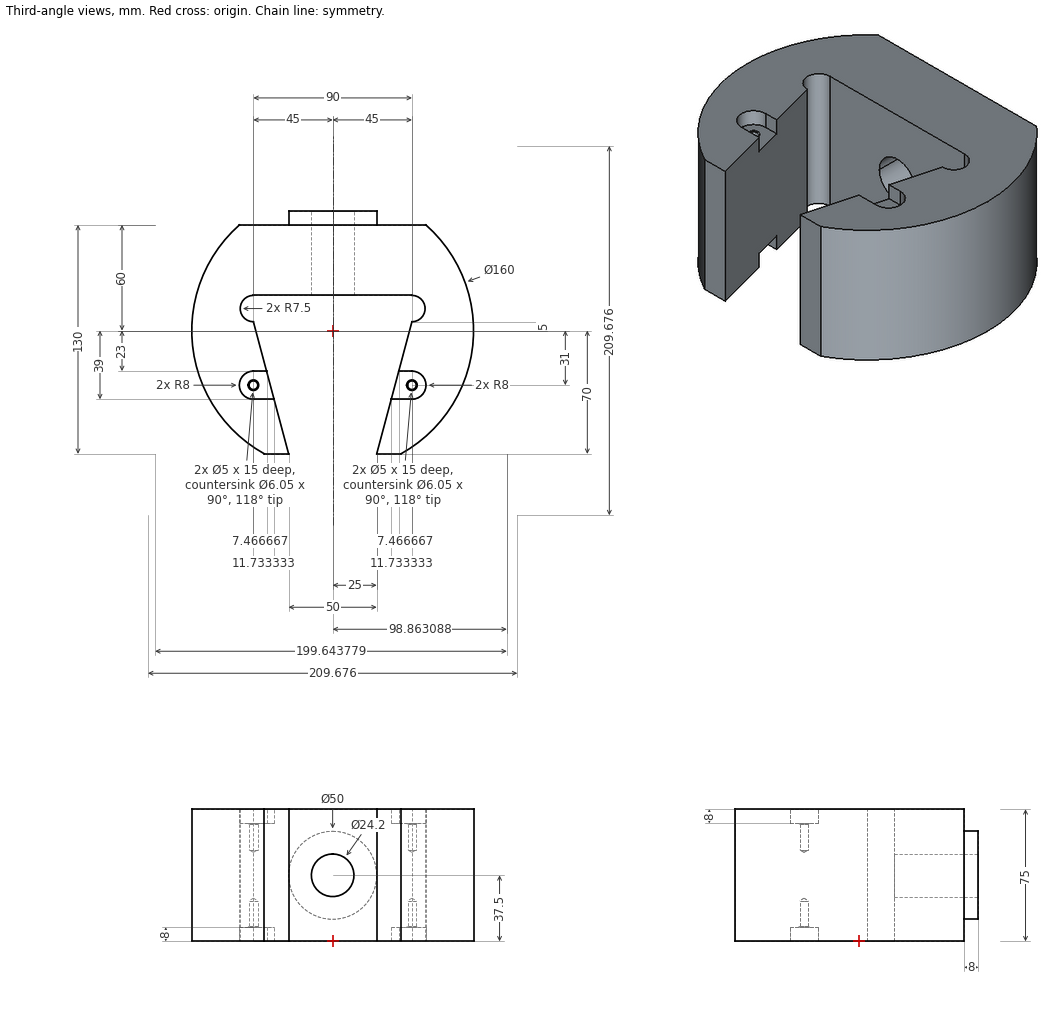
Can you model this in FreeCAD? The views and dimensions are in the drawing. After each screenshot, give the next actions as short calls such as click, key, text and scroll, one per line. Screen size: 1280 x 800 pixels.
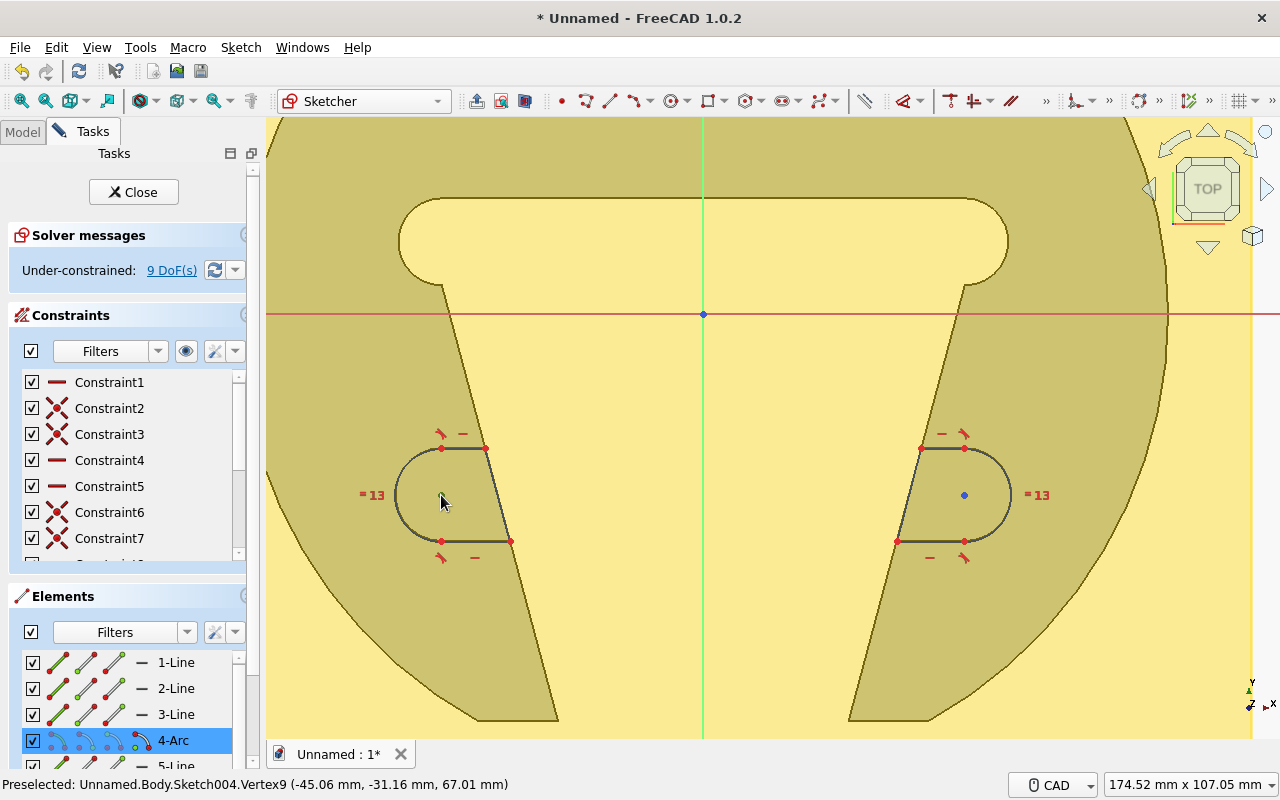
click(964, 495)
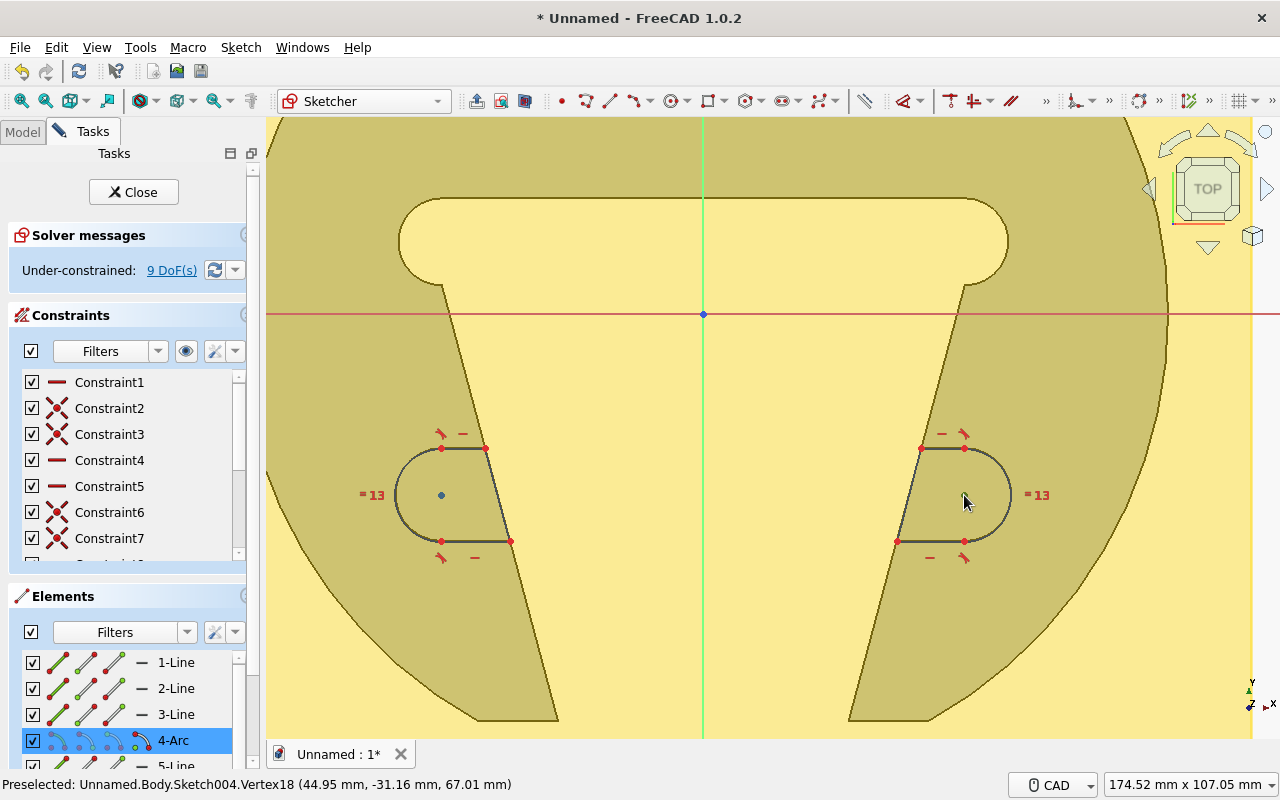
click(703, 671)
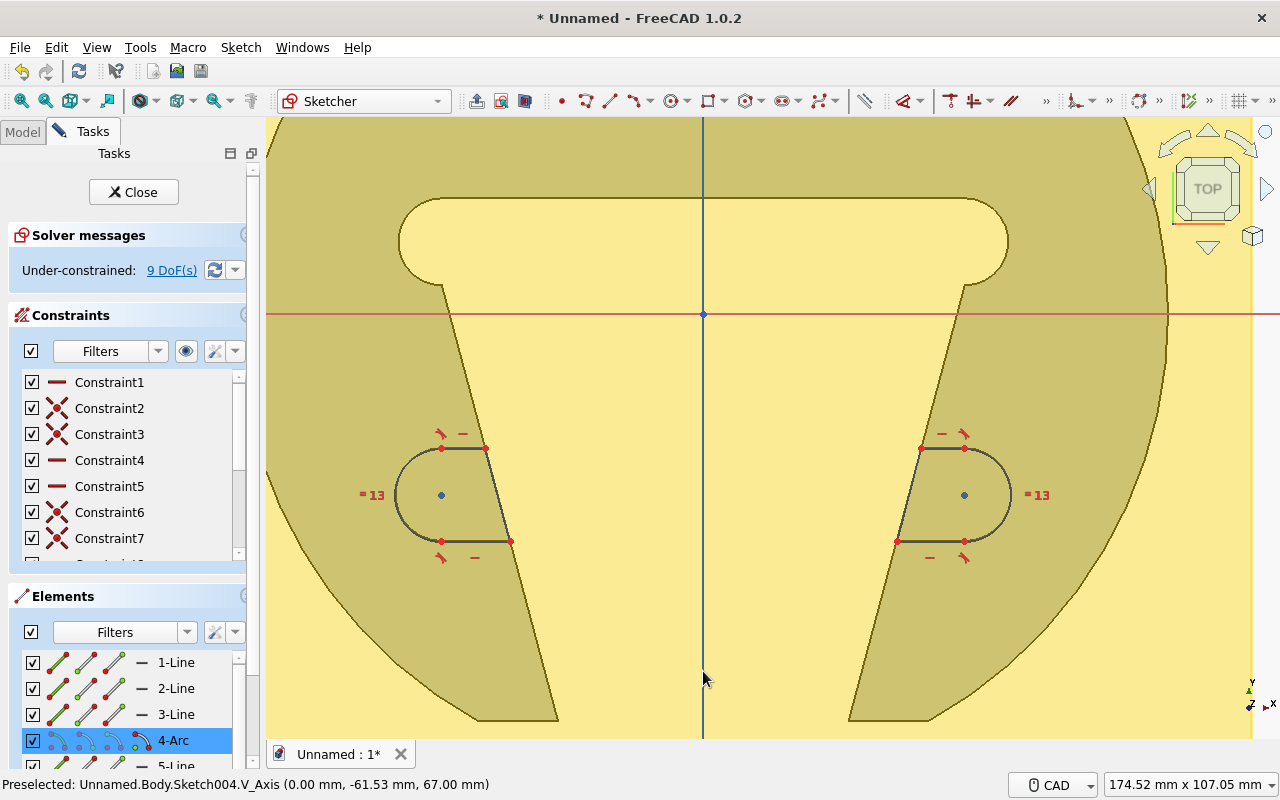
key(s)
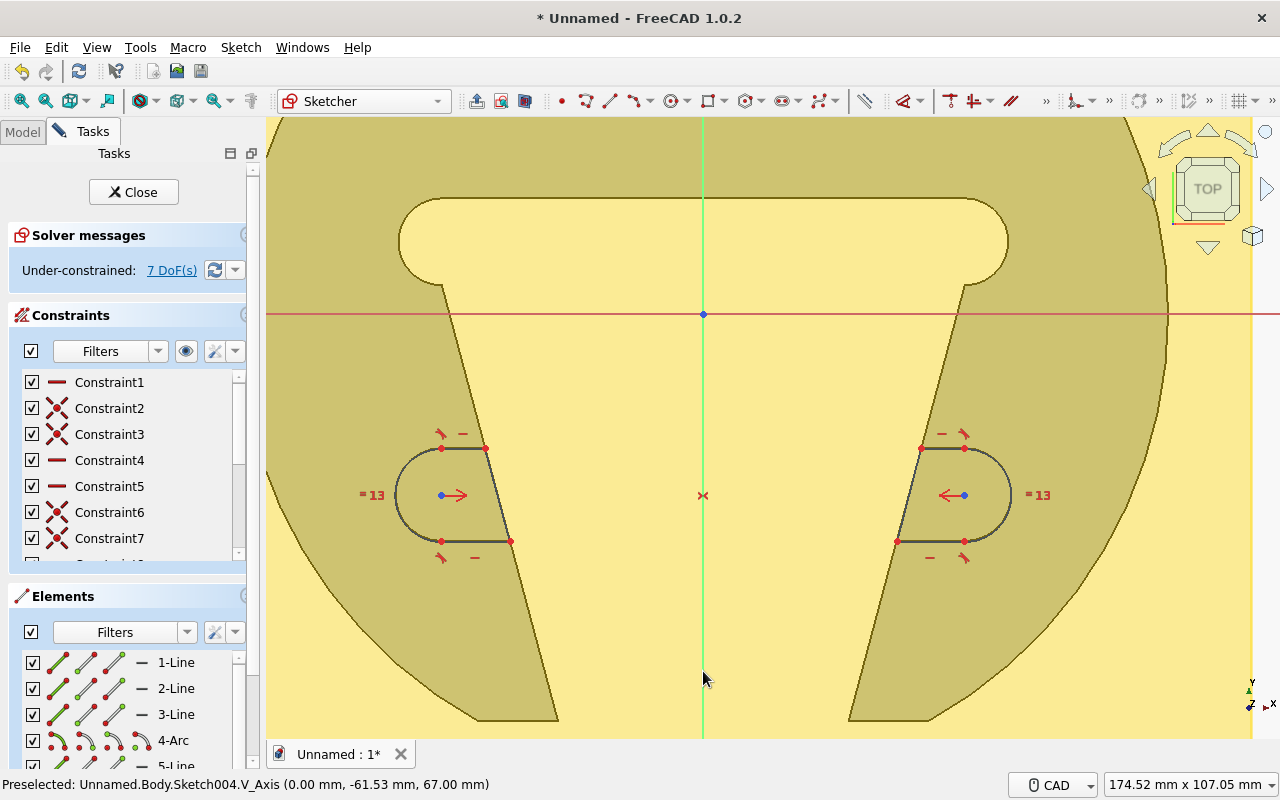
key(d)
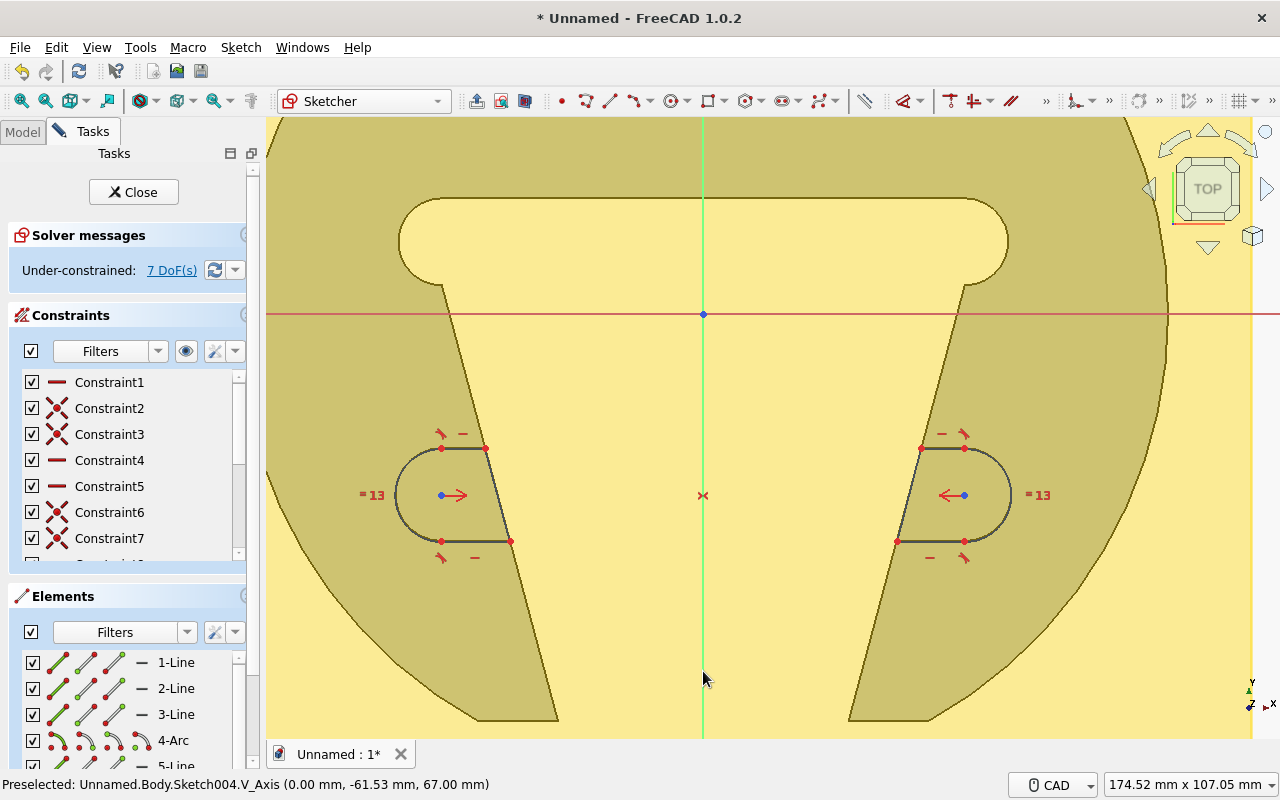
click(404, 468)
click(378, 449)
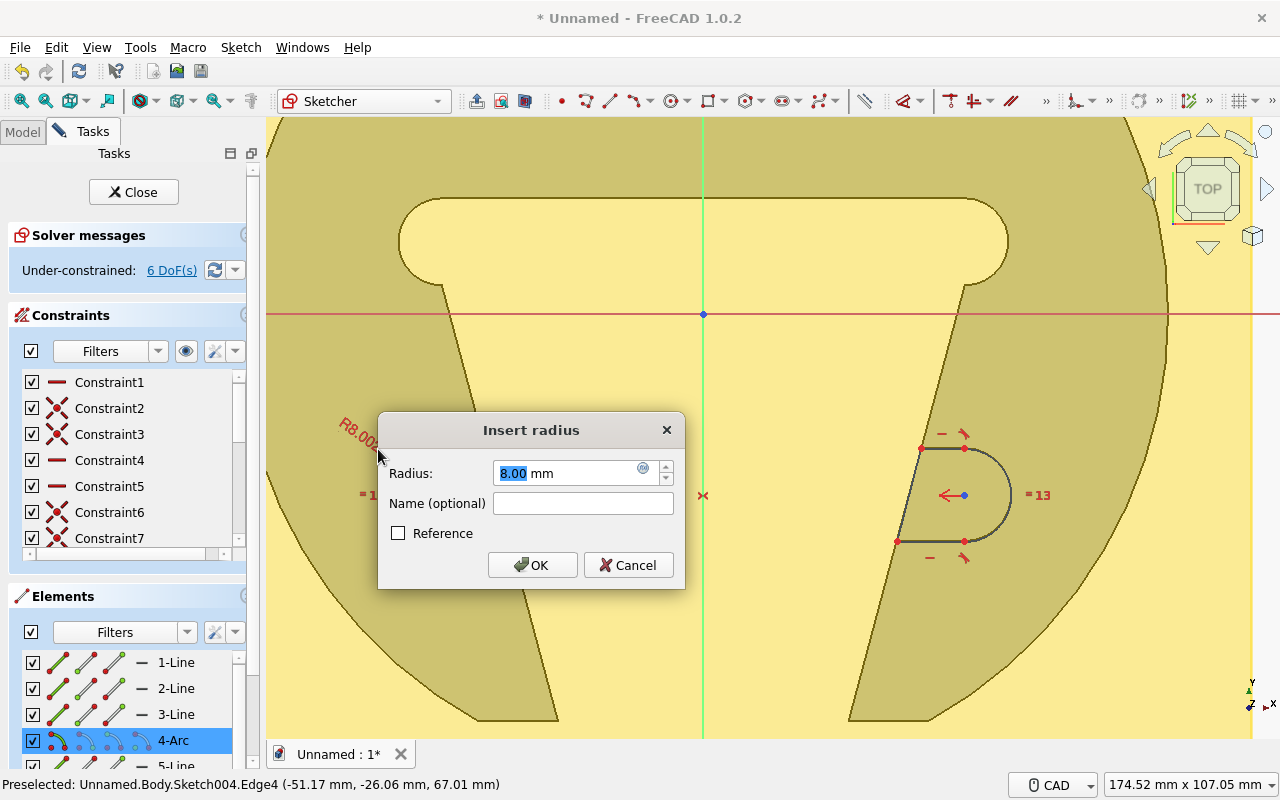
text(8)
key(Return)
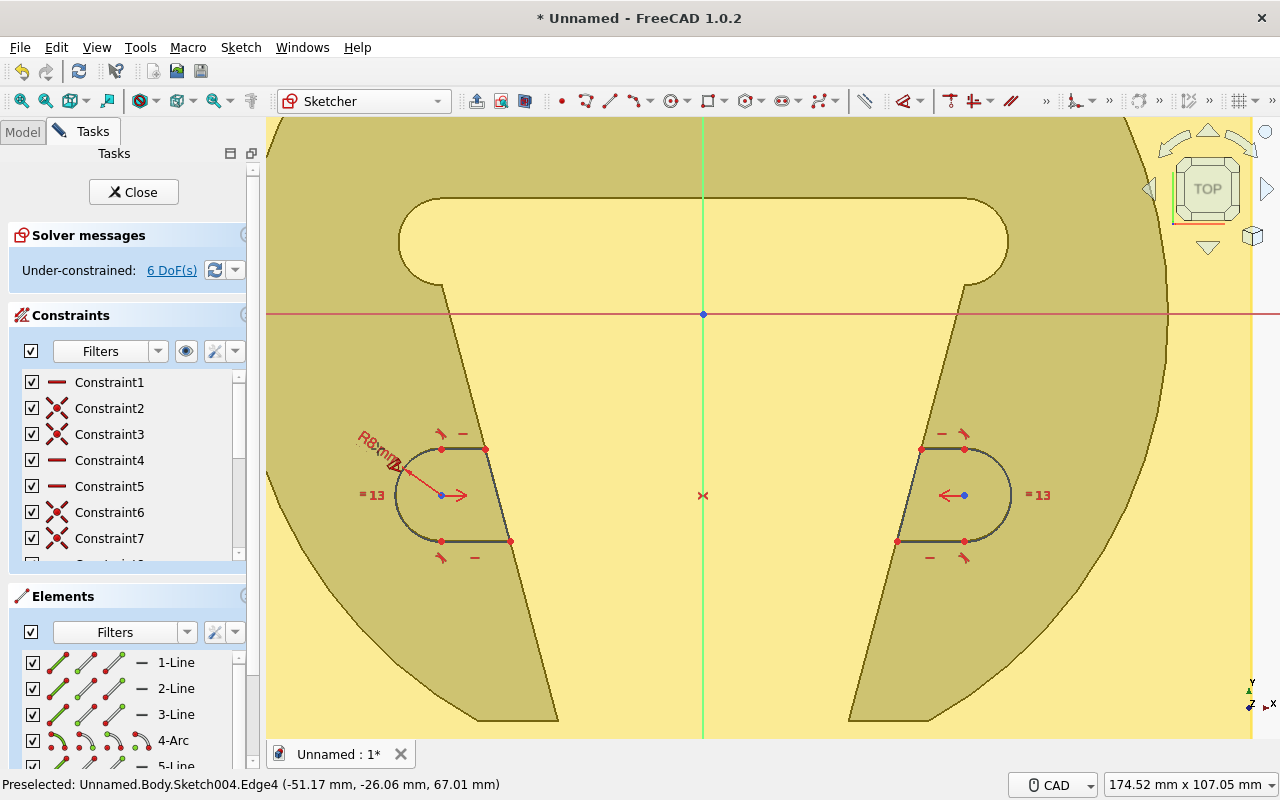
click(442, 449)
click(573, 280)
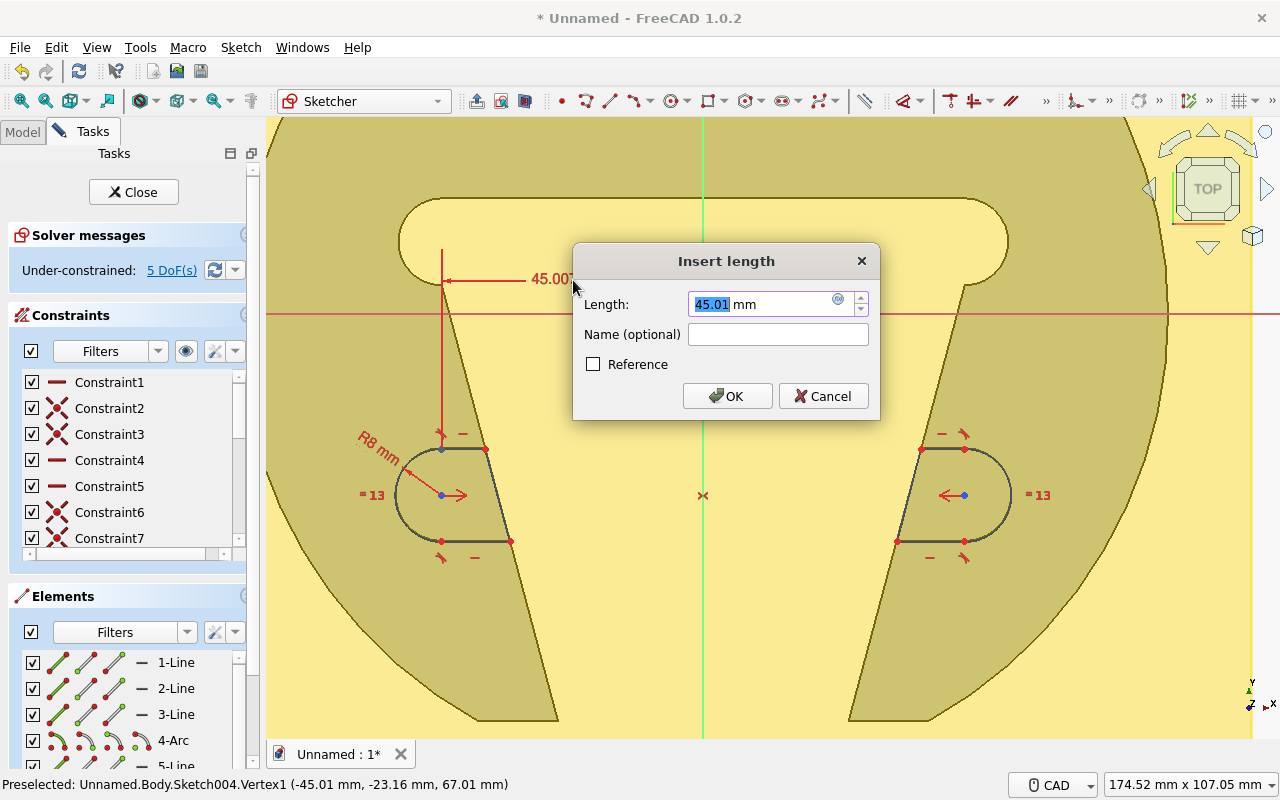
text(45)
key(Return)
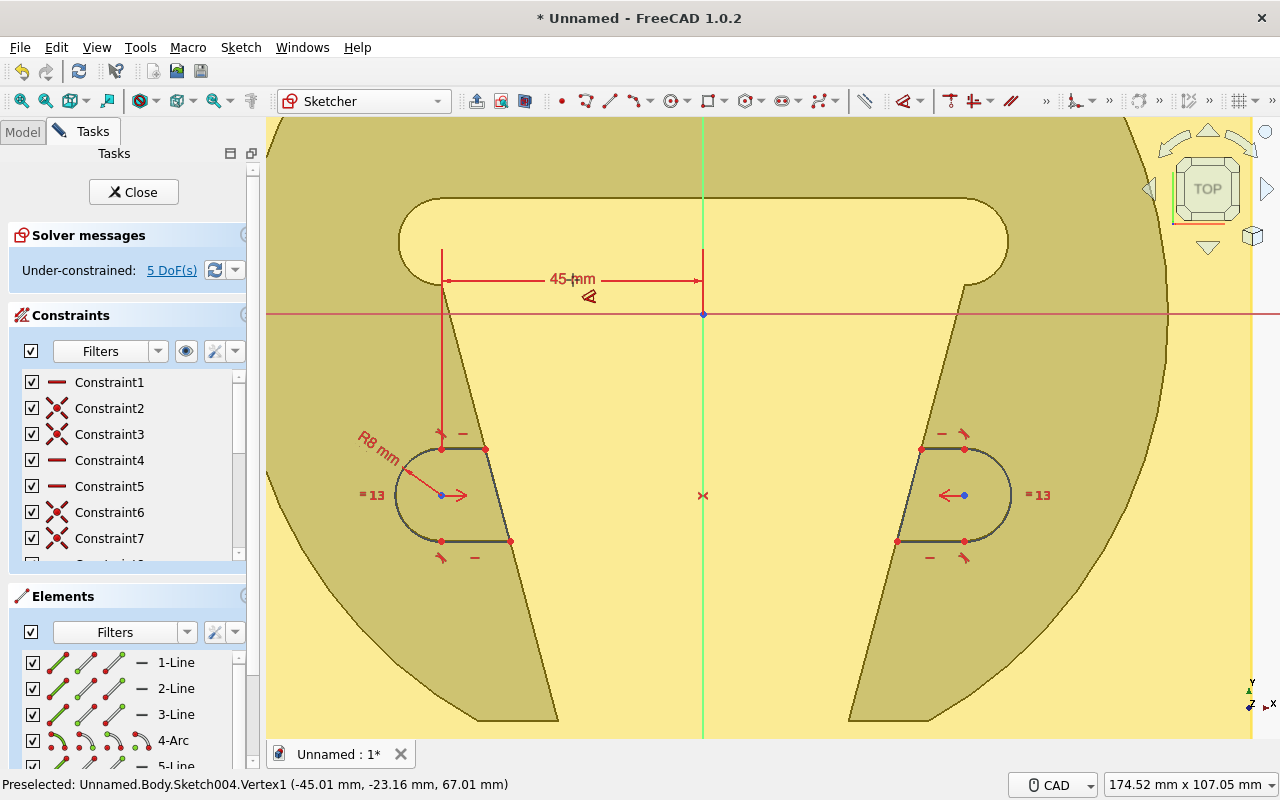
click(442, 449)
click(408, 382)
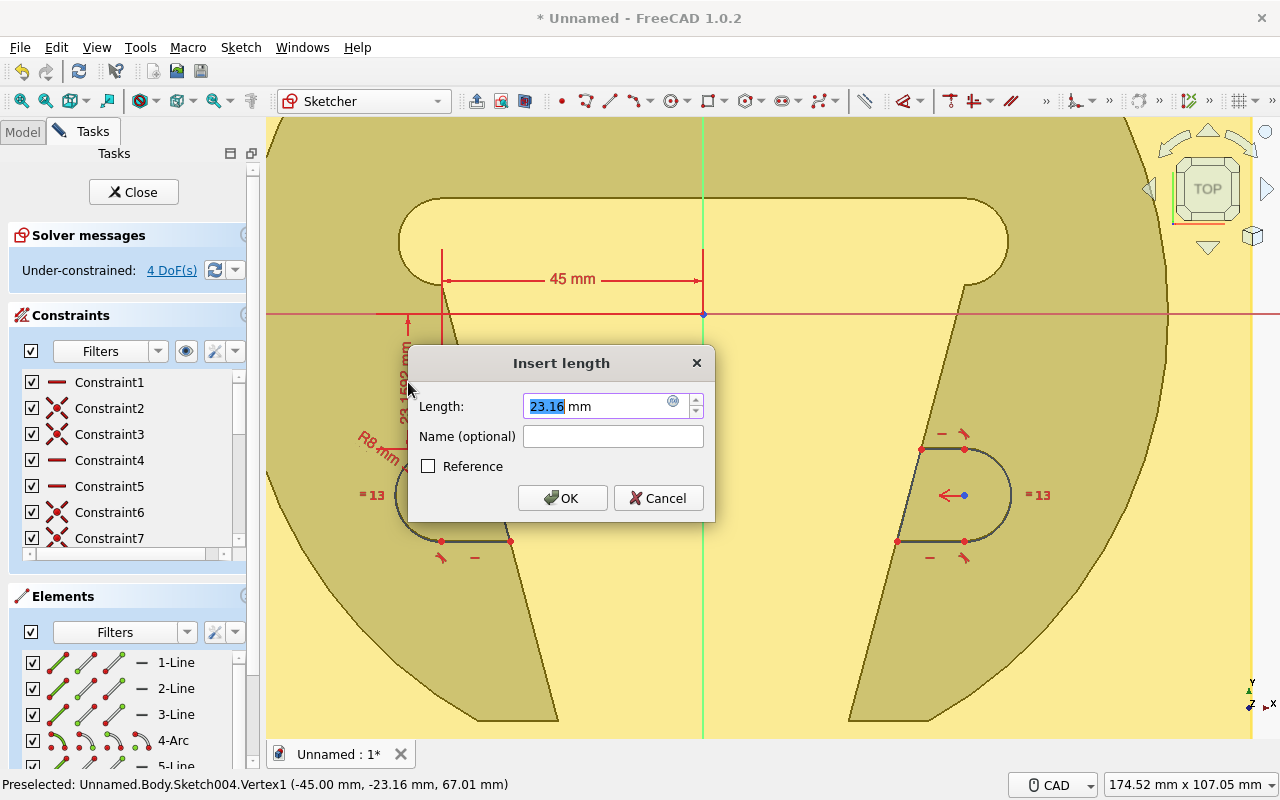
text(23)
key(Return)